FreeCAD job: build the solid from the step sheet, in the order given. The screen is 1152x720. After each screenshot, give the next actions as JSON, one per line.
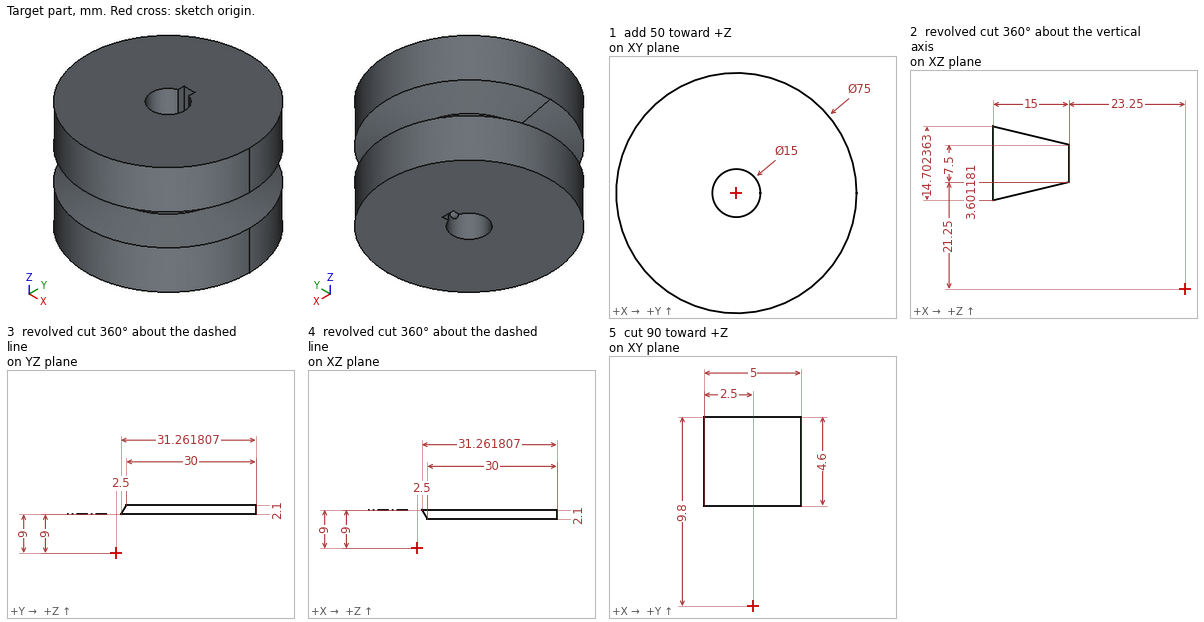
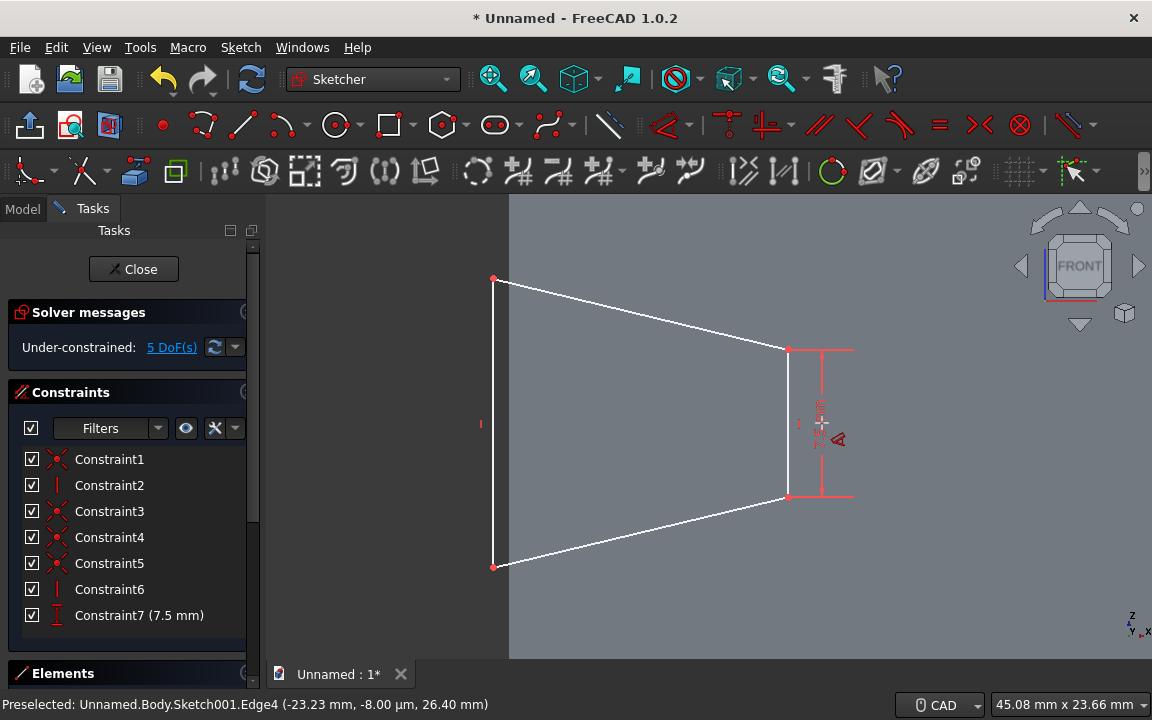
{"action": "left_click", "coordinate": [699, 519]}
{"action": "left_click", "coordinate": [640, 602]}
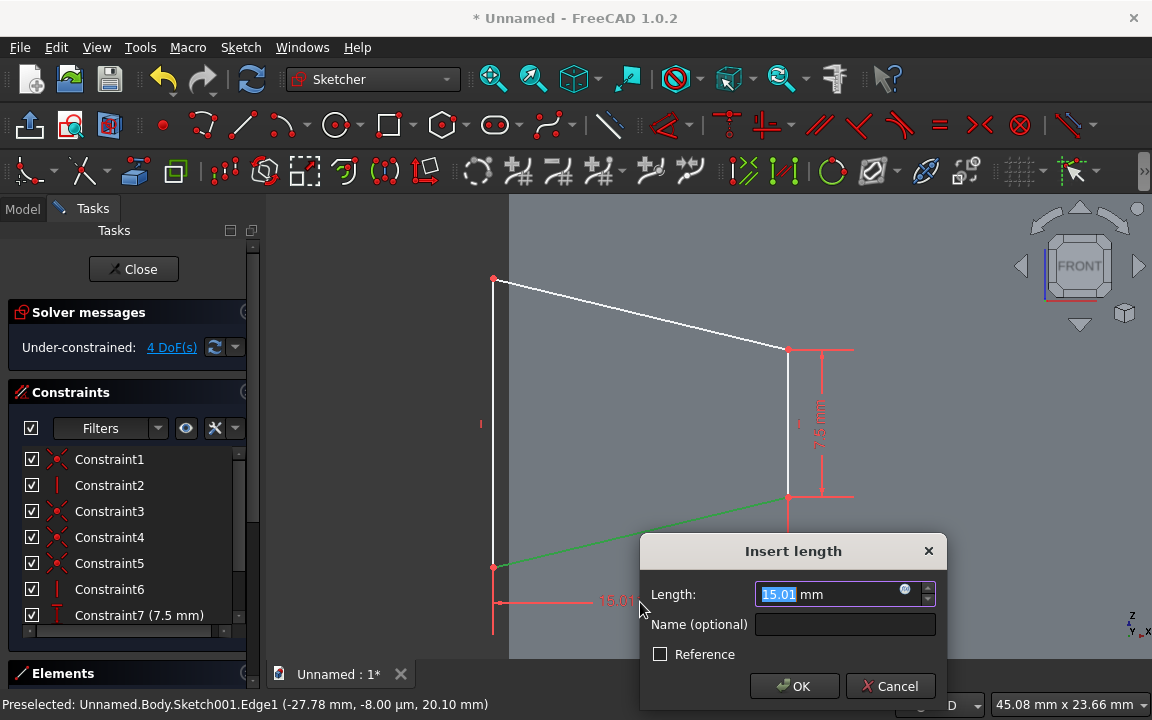
{"action": "type", "text": "15"}
{"action": "key", "text": "Return"}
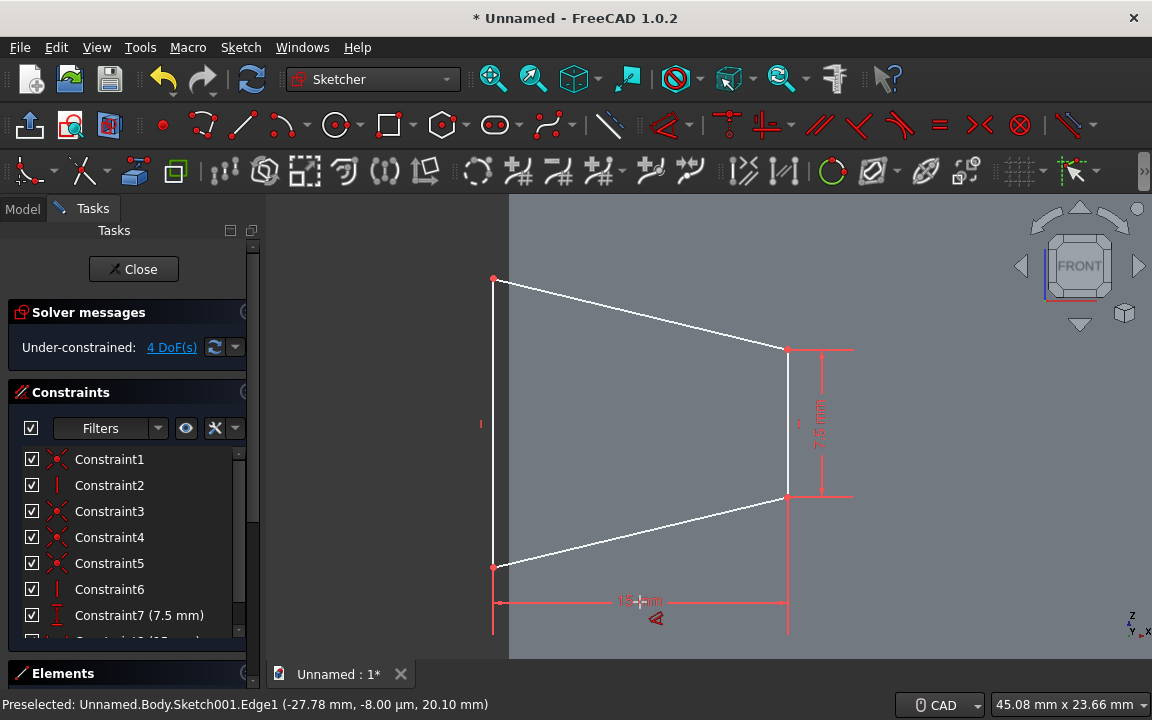
{"action": "left_click", "coordinate": [788, 497]}
{"action": "left_click", "coordinate": [887, 463]}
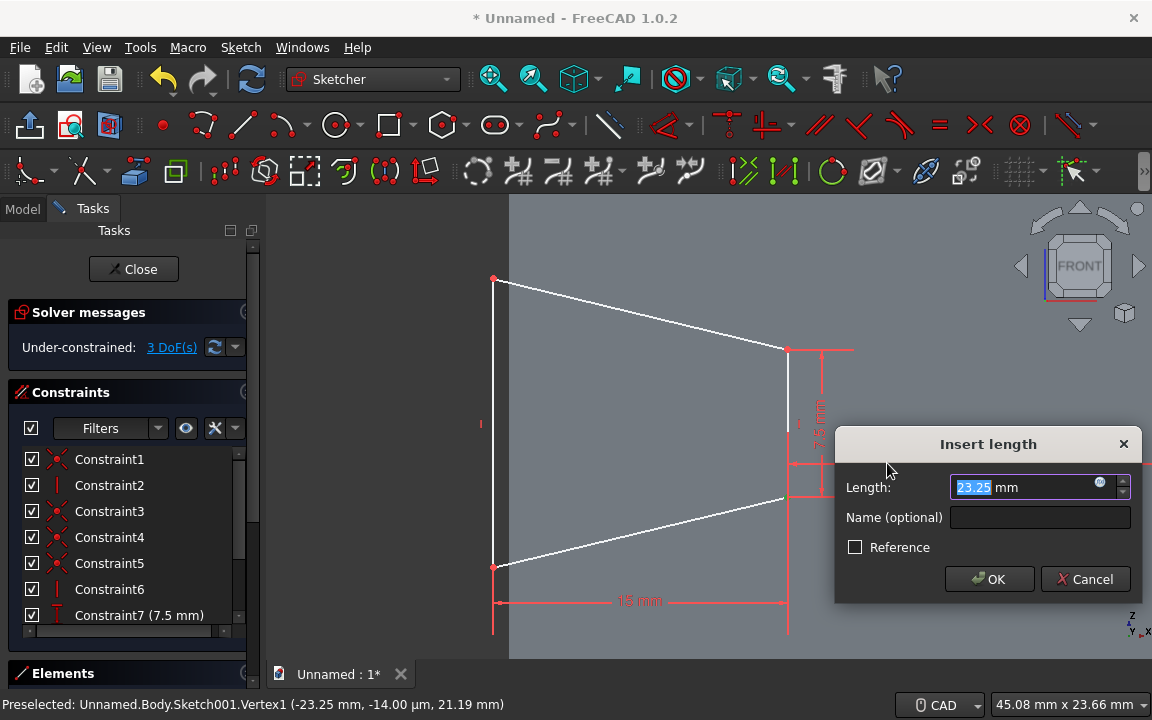
{"action": "type", "text": "23.25"}
{"action": "key", "text": "Return"}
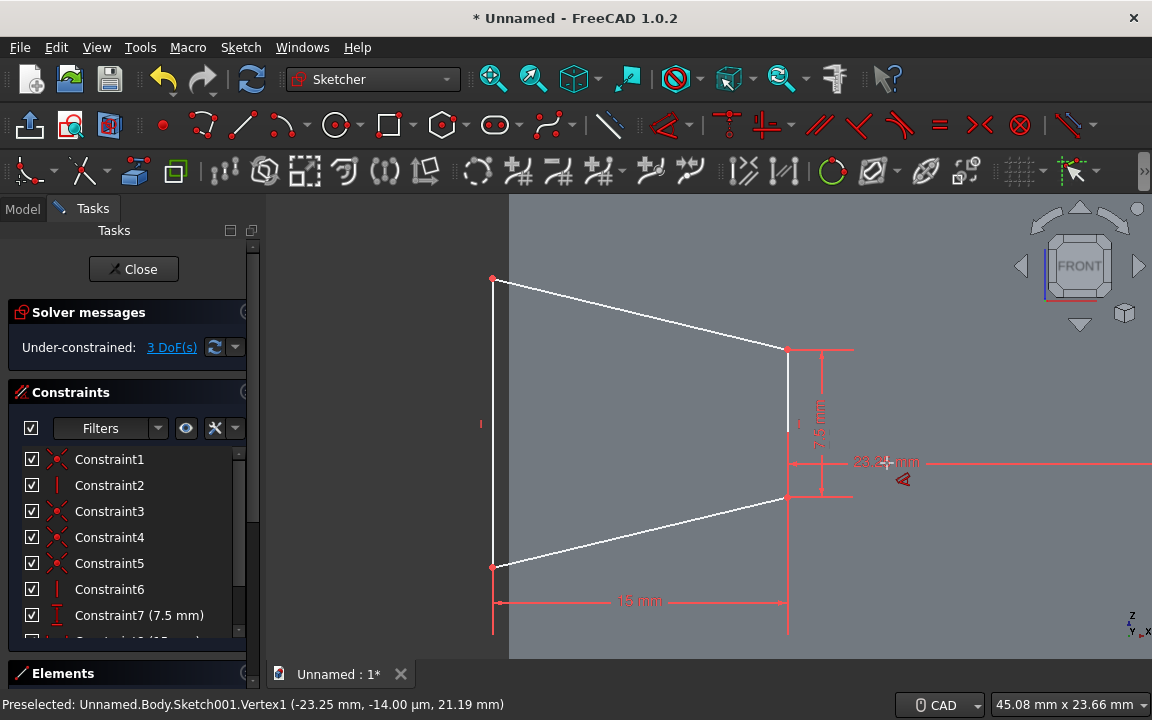
{"action": "left_click", "coordinate": [788, 497]}
{"action": "left_click", "coordinate": [754, 564]}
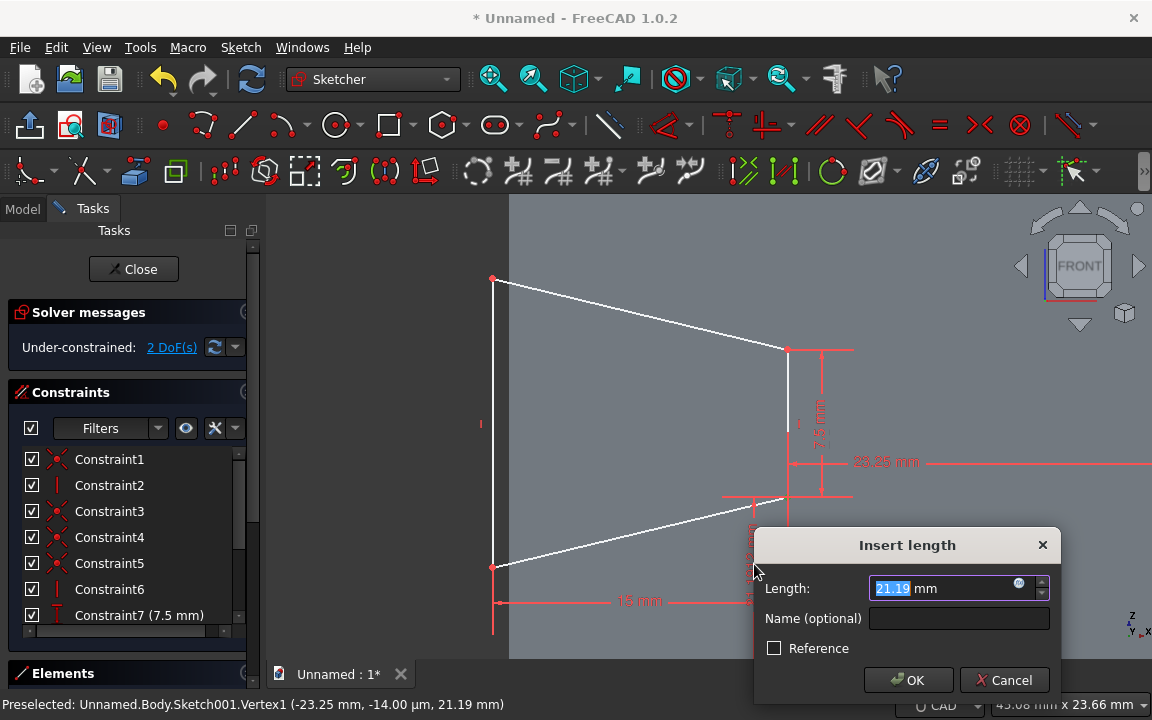
{"action": "type", "text": "21.25"}
{"action": "key", "text": "Return"}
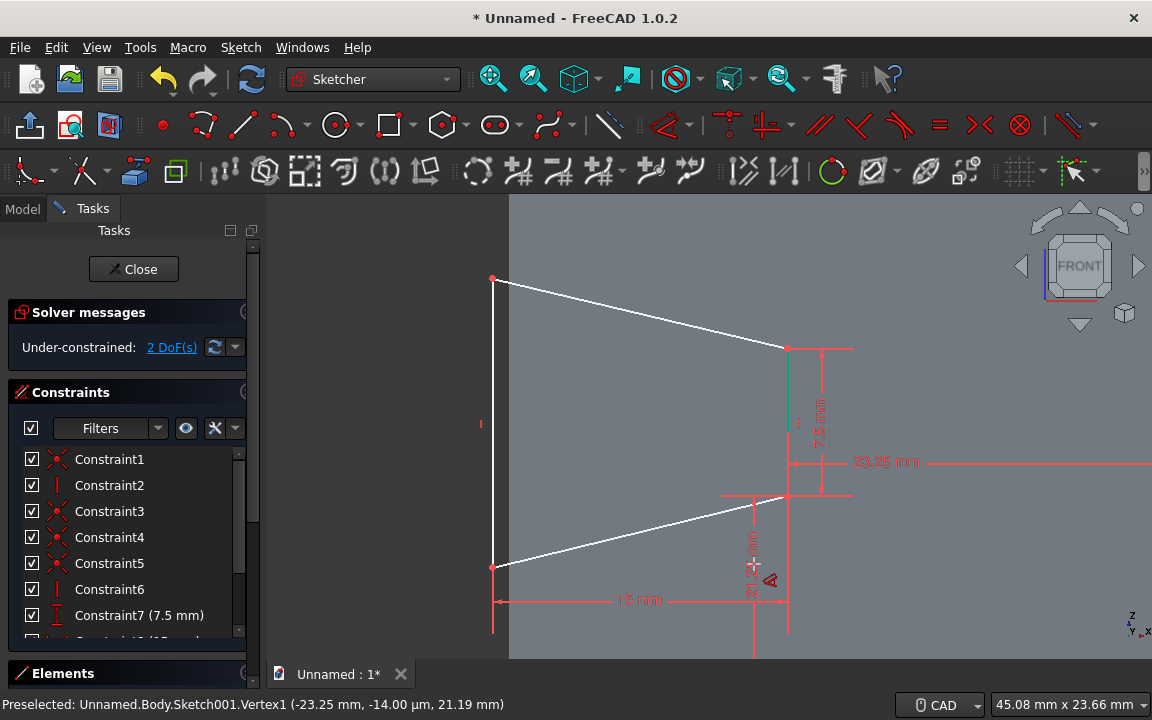
{"action": "left_click", "coordinate": [493, 481]}
{"action": "left_click", "coordinate": [459, 424]}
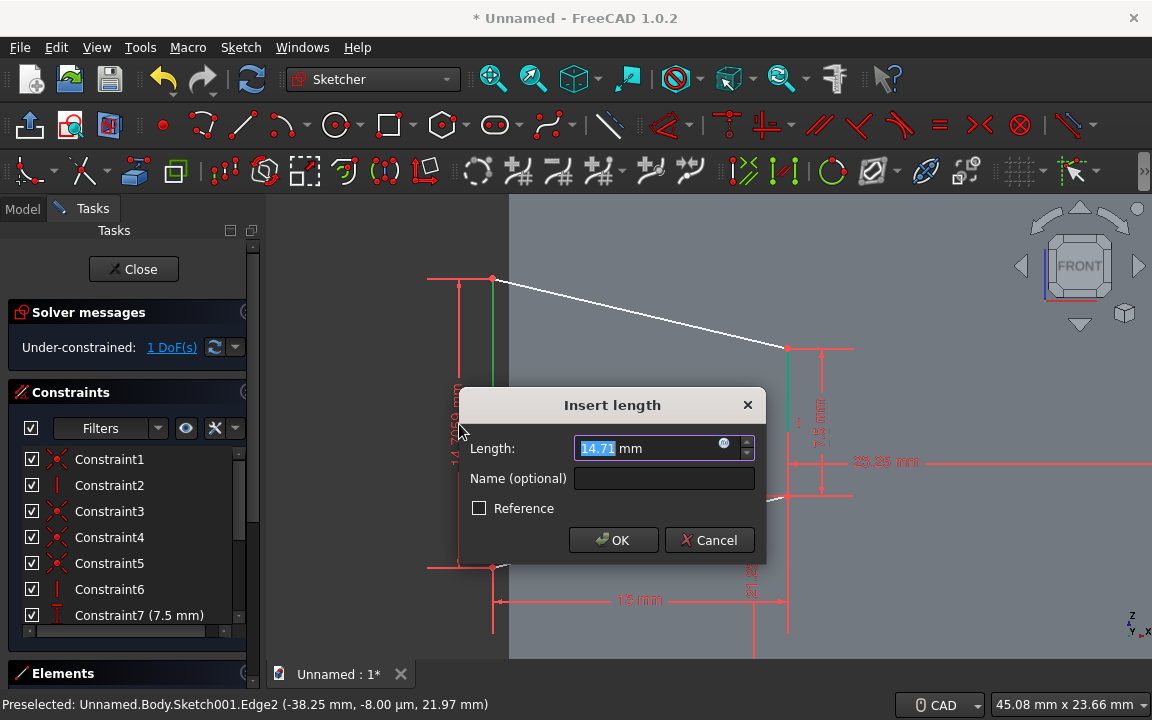
{"action": "type", "text": "14.702363"}
{"action": "key", "text": "Return"}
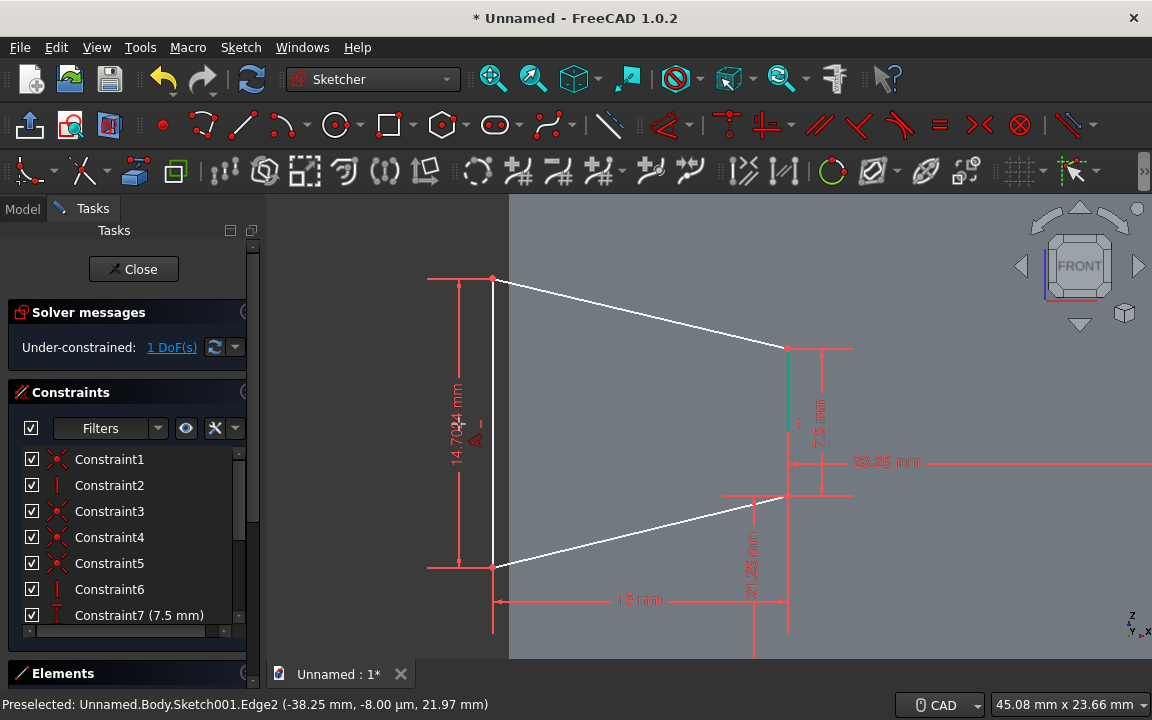
{"action": "left_click", "coordinate": [699, 518]}
{"action": "left_click", "coordinate": [459, 532]}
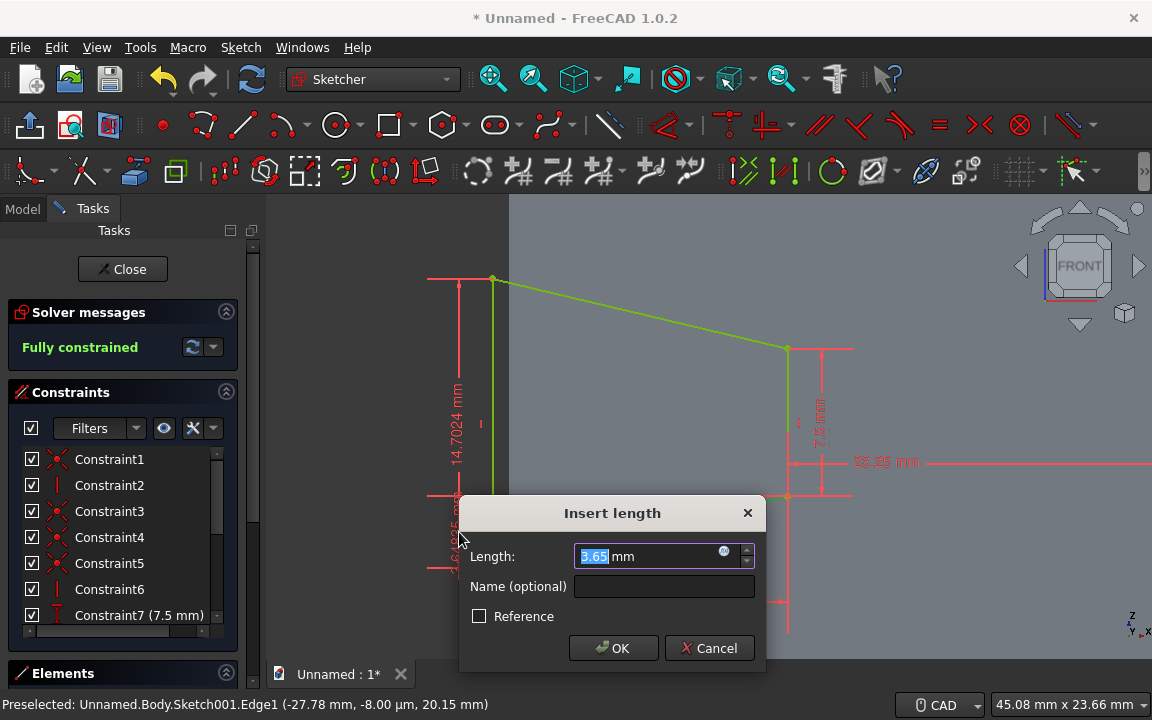
{"action": "type", "text": "3.601181"}
{"action": "key", "text": "Return"}
{"action": "key", "text": "Escape"}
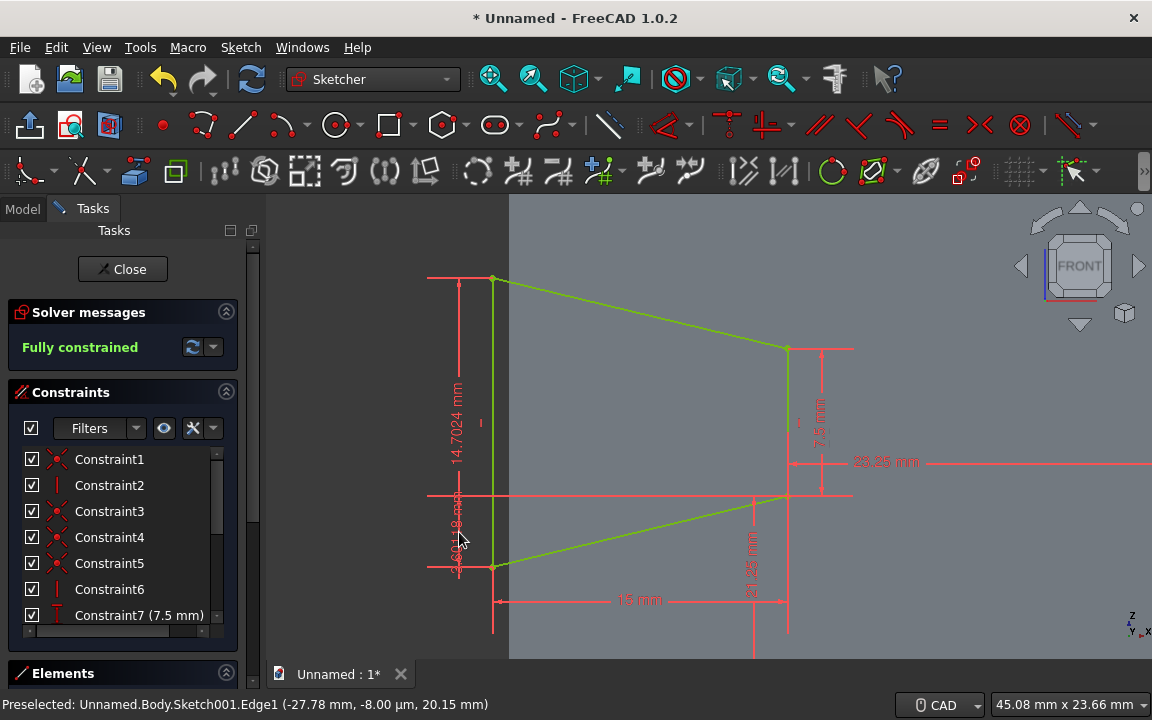
{"action": "left_click", "coordinate": [123, 269]}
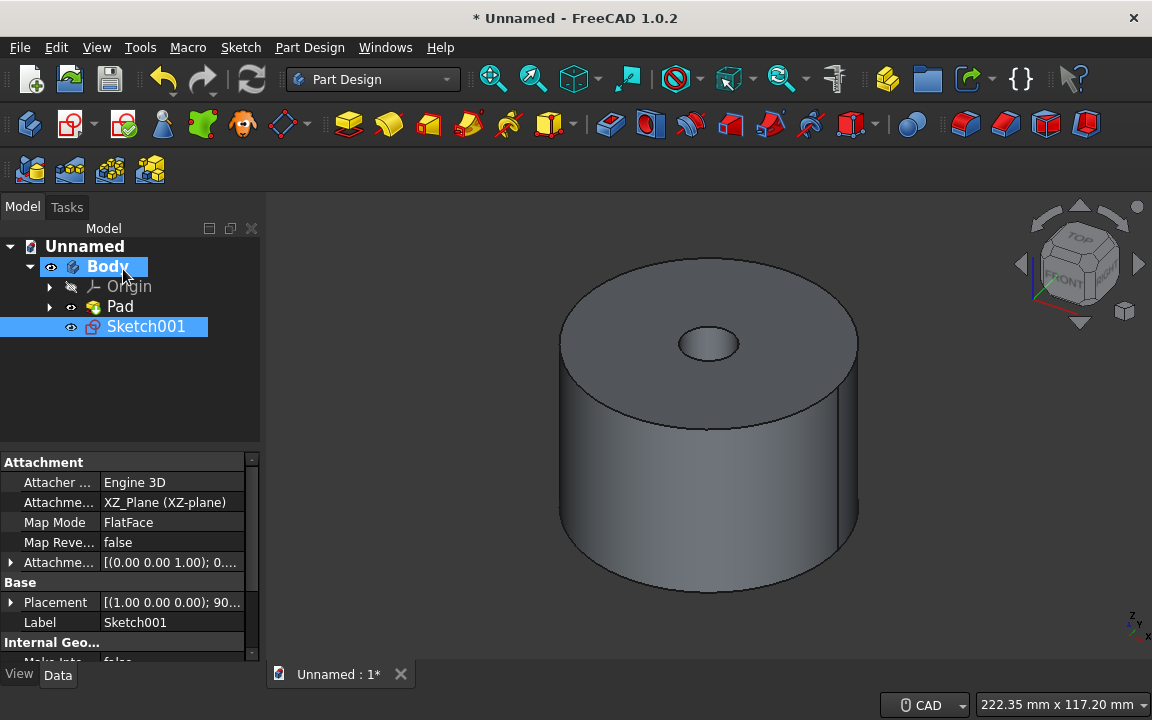
{"action": "left_click", "coordinate": [692, 124]}